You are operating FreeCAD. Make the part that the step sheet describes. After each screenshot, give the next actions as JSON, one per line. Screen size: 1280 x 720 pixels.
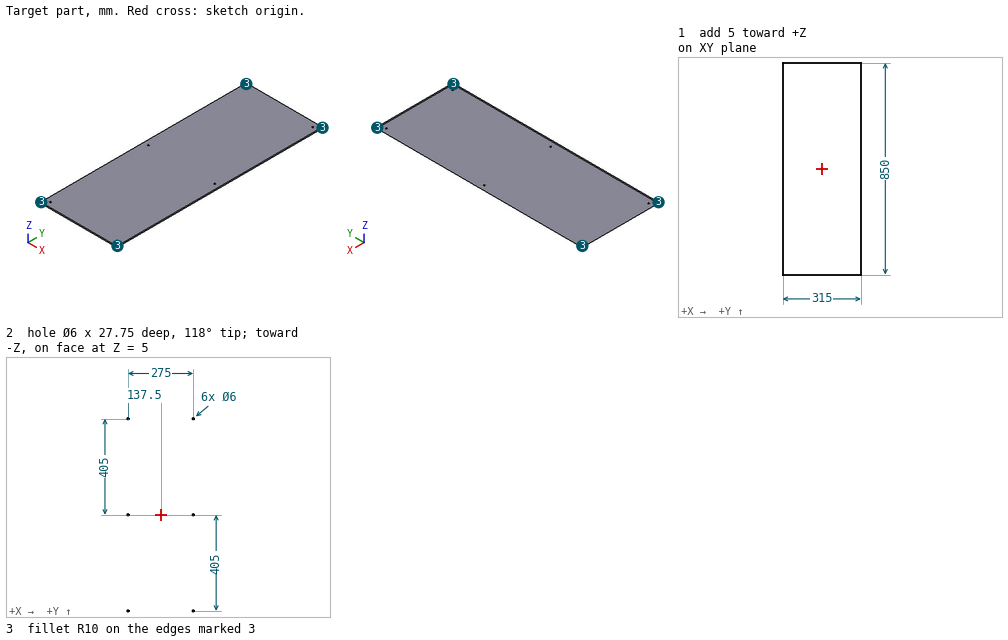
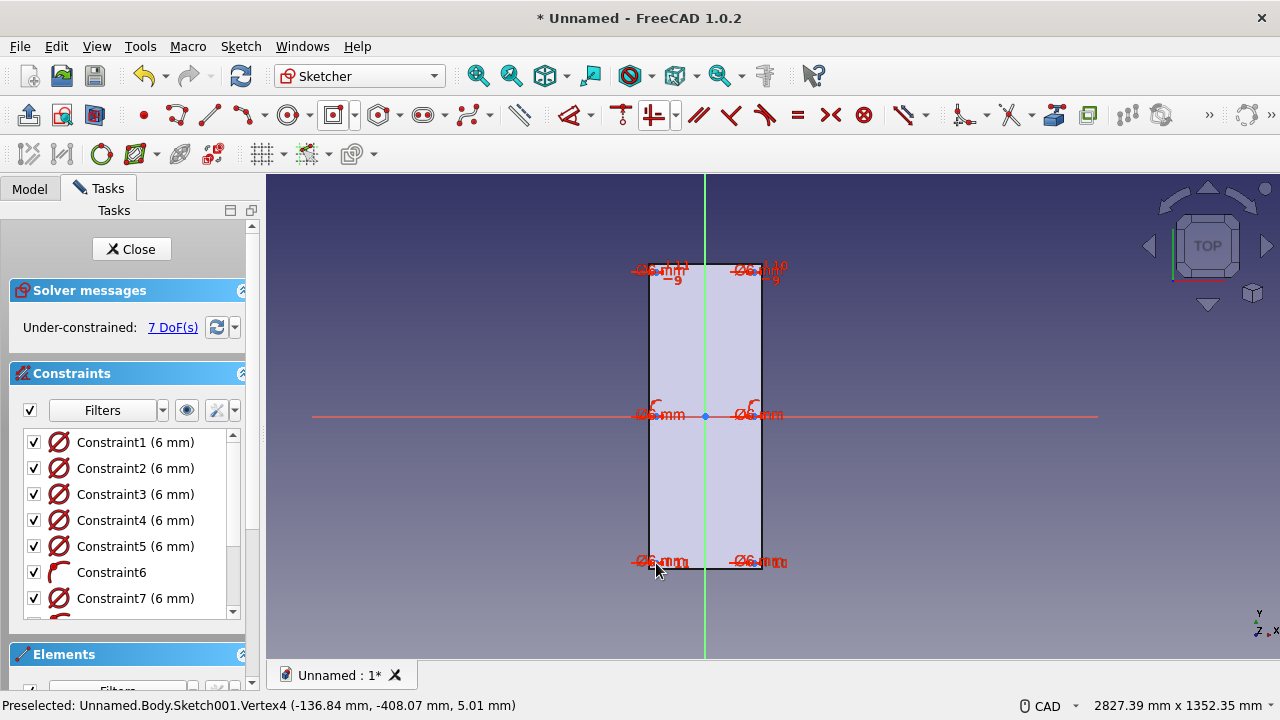
{"action": "left_click", "coordinate": [754, 563]}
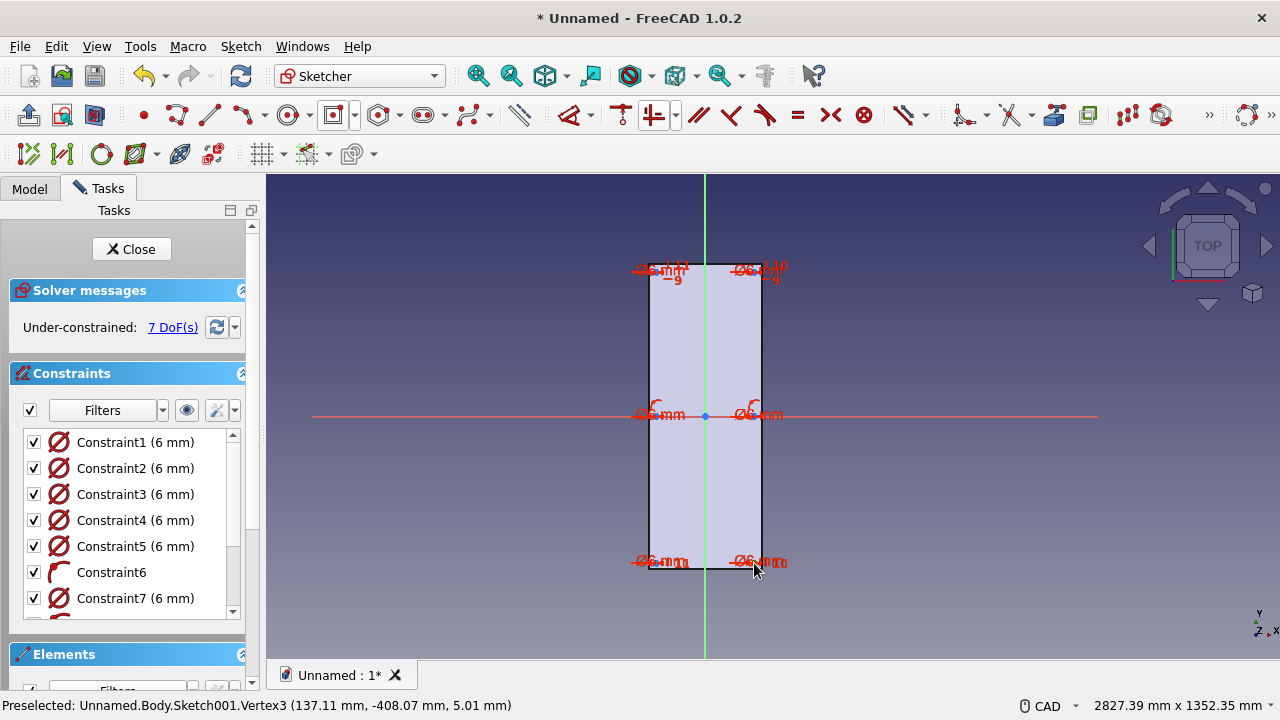
{"action": "left_click", "coordinate": [656, 563]}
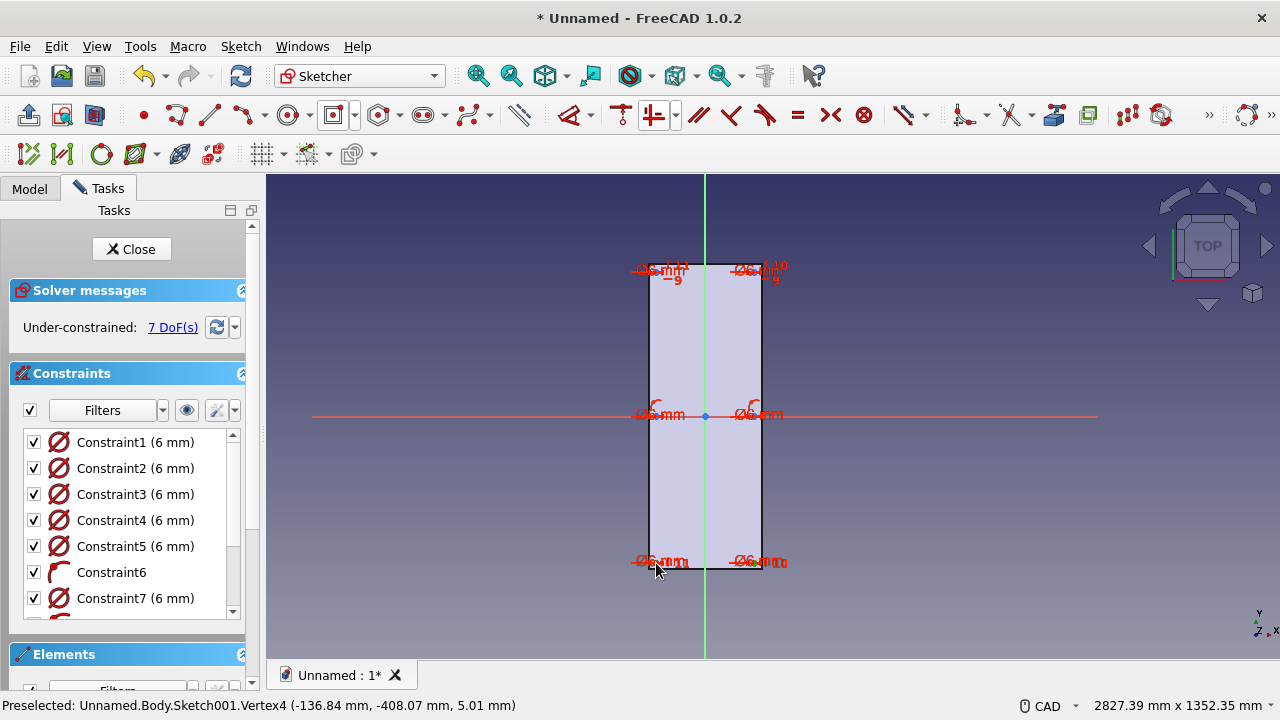
{"action": "left_click", "coordinate": [676, 116]}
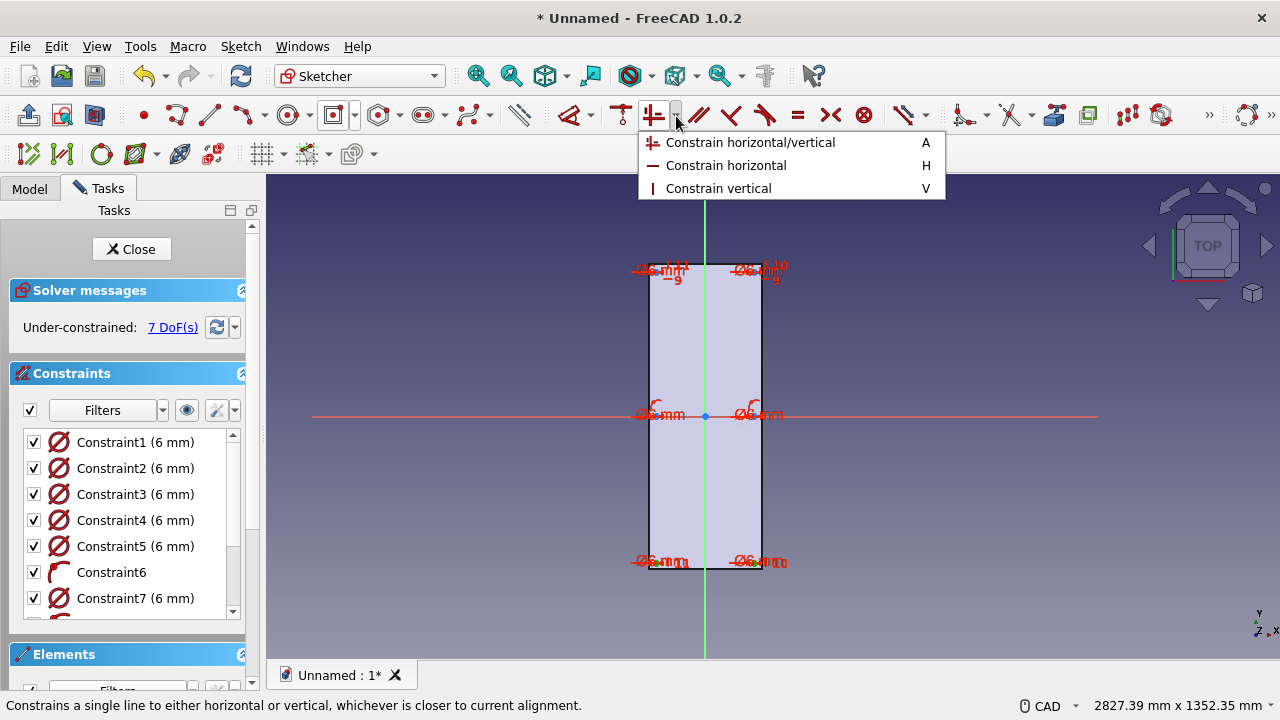
{"action": "left_click", "coordinate": [792, 166]}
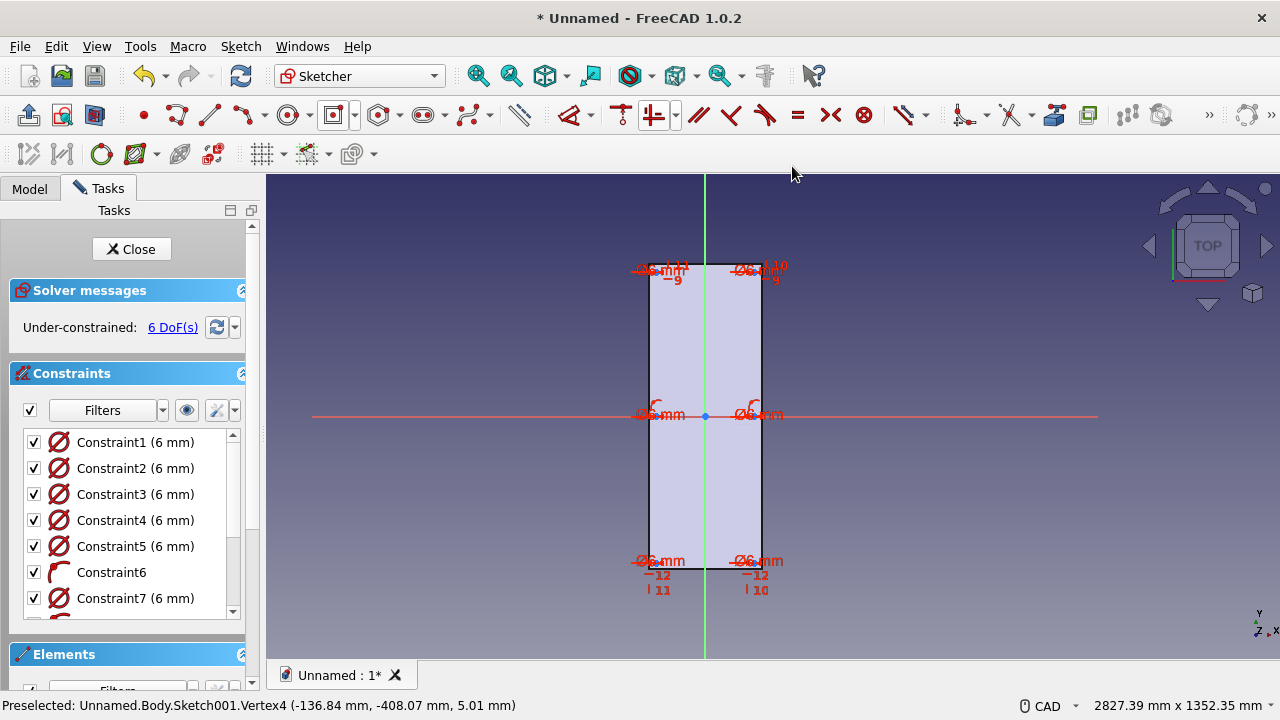
{"action": "left_click", "coordinate": [656, 272]}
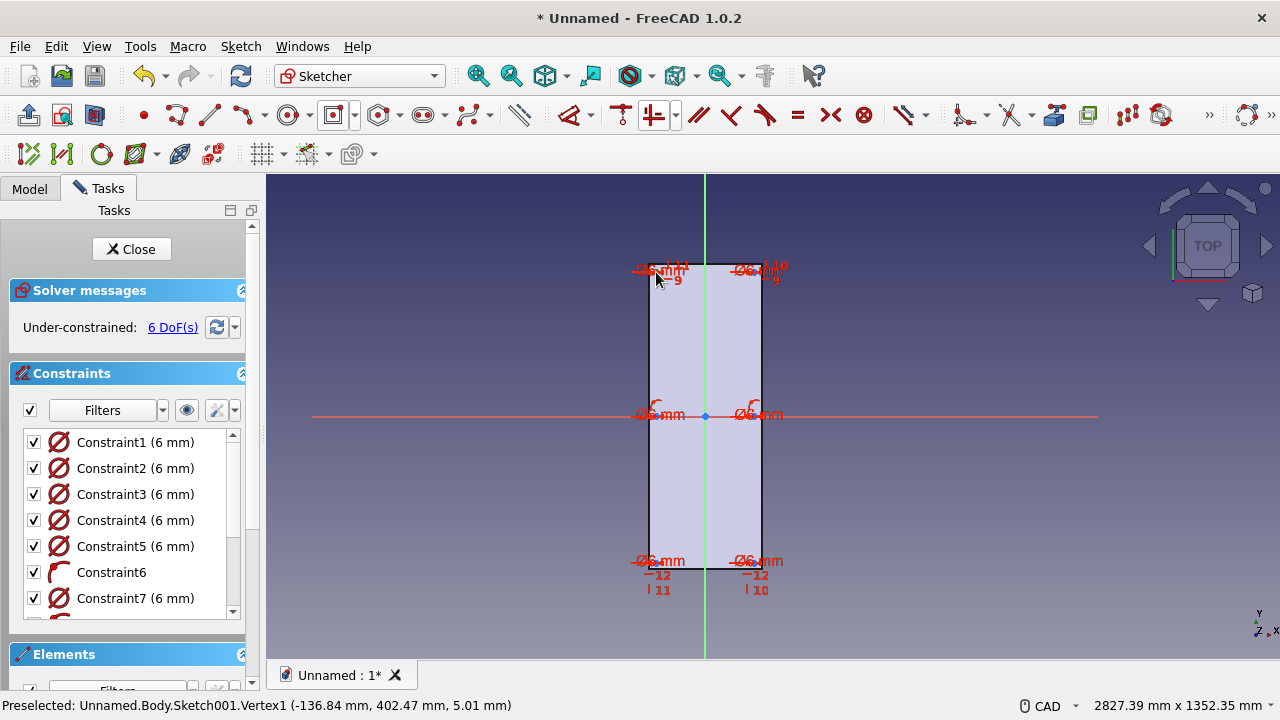
{"action": "left_click", "coordinate": [656, 417]}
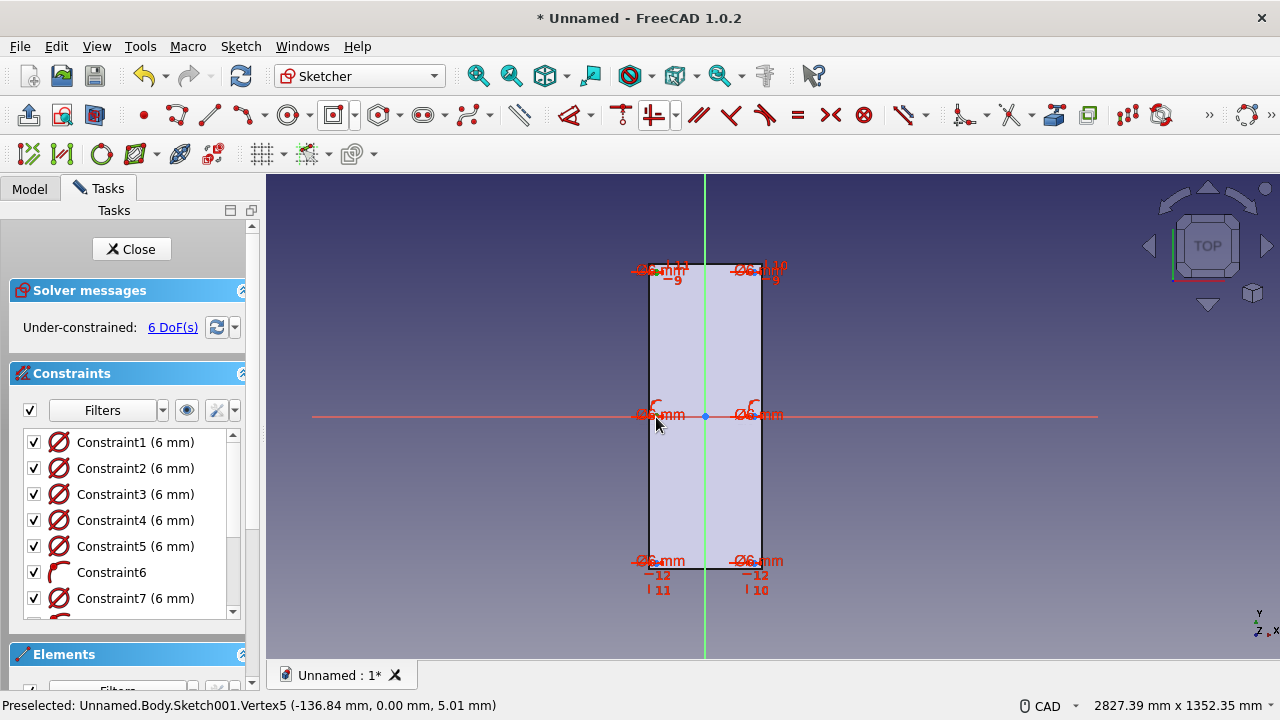
{"action": "left_click", "coordinate": [676, 116]}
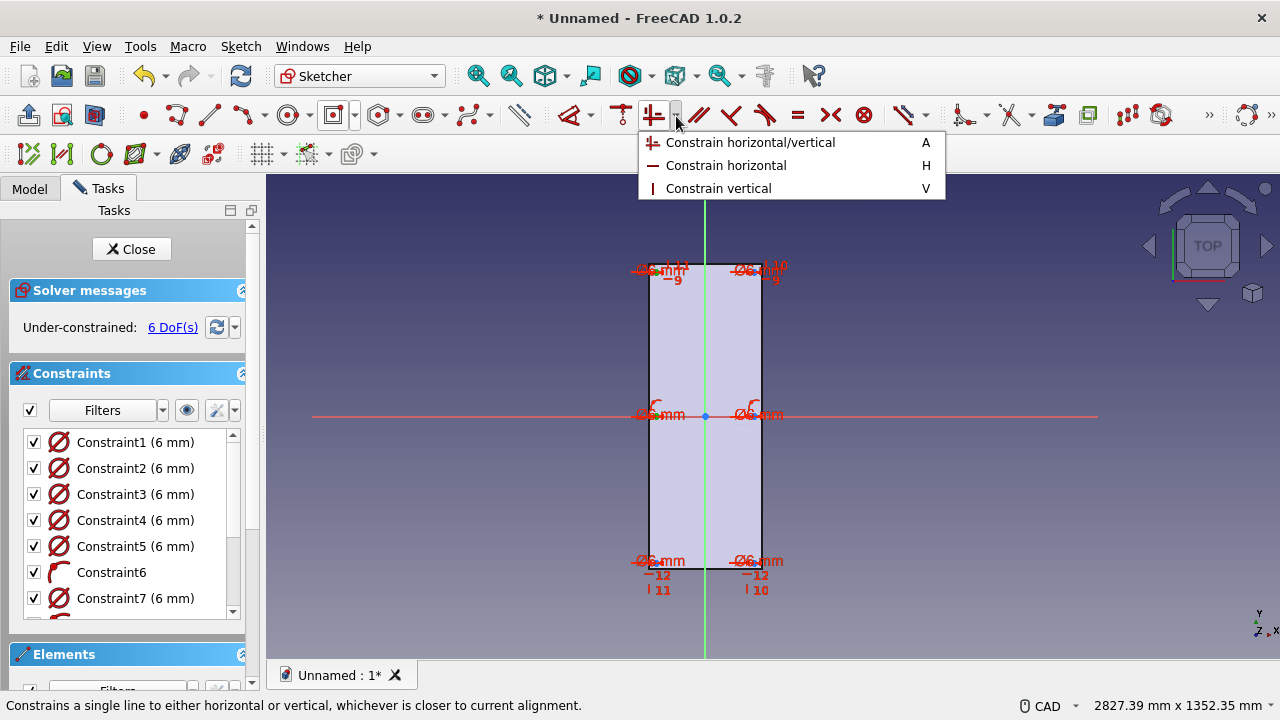
{"action": "left_click", "coordinate": [792, 188]}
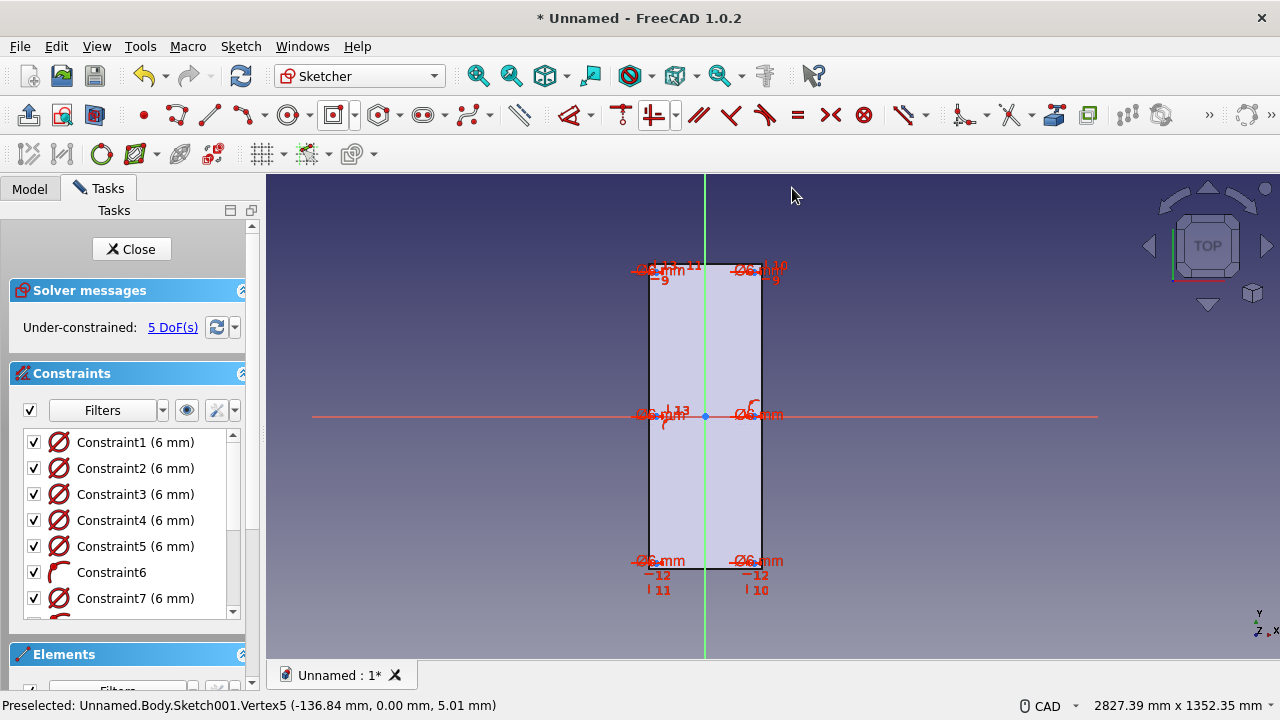
{"action": "left_click", "coordinate": [754, 272]}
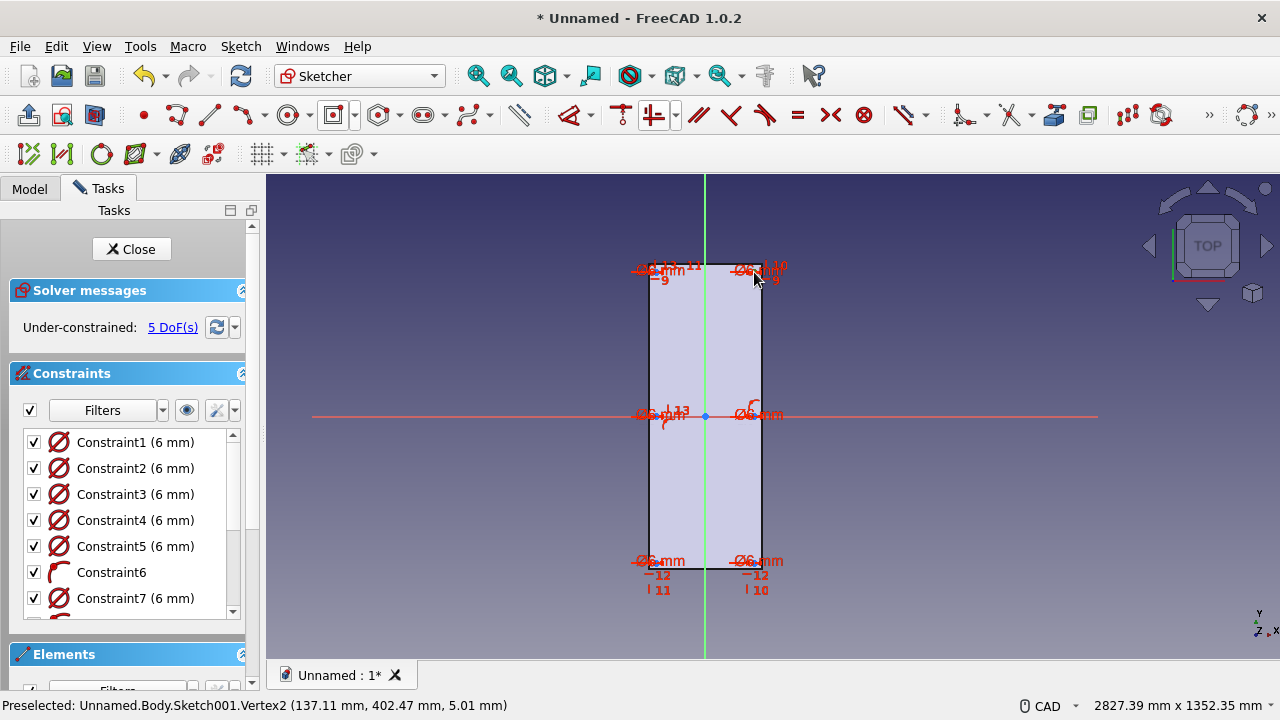
{"action": "left_click", "coordinate": [755, 417]}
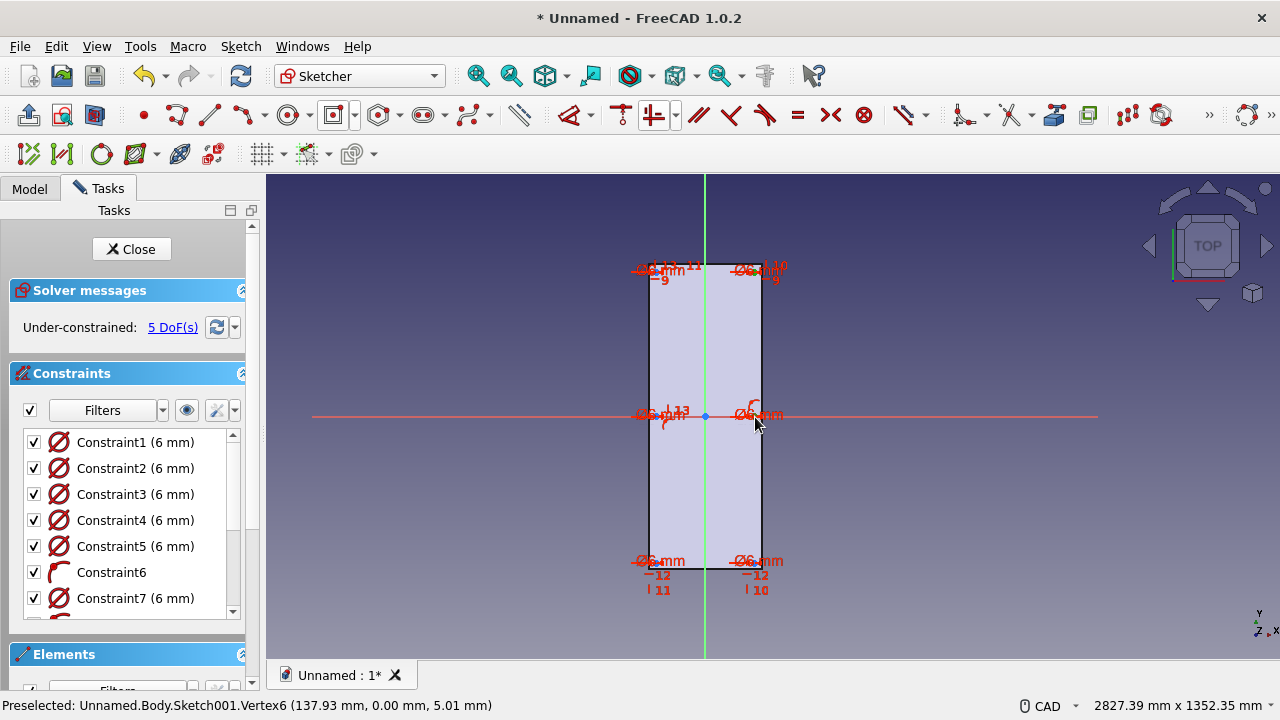
{"action": "left_click", "coordinate": [676, 116]}